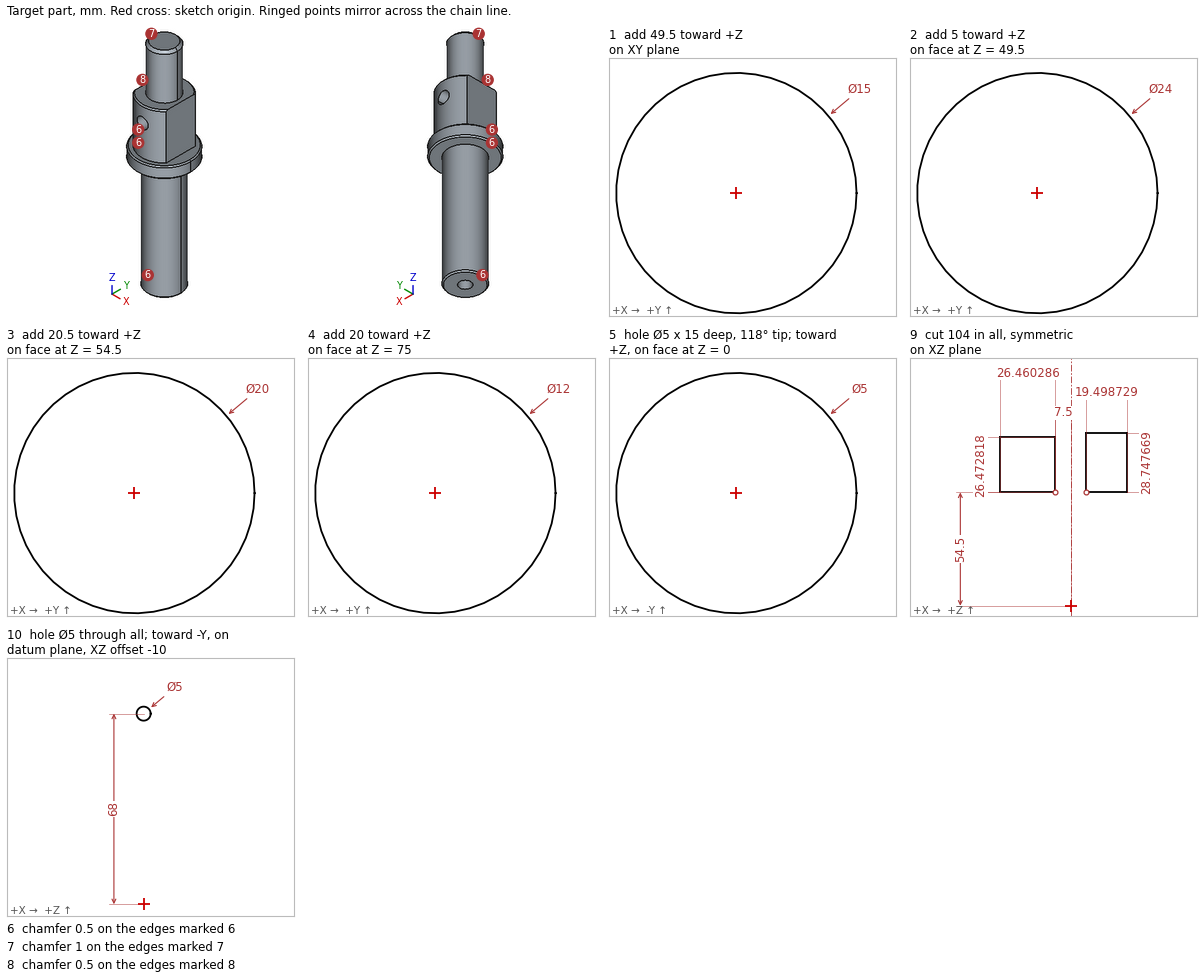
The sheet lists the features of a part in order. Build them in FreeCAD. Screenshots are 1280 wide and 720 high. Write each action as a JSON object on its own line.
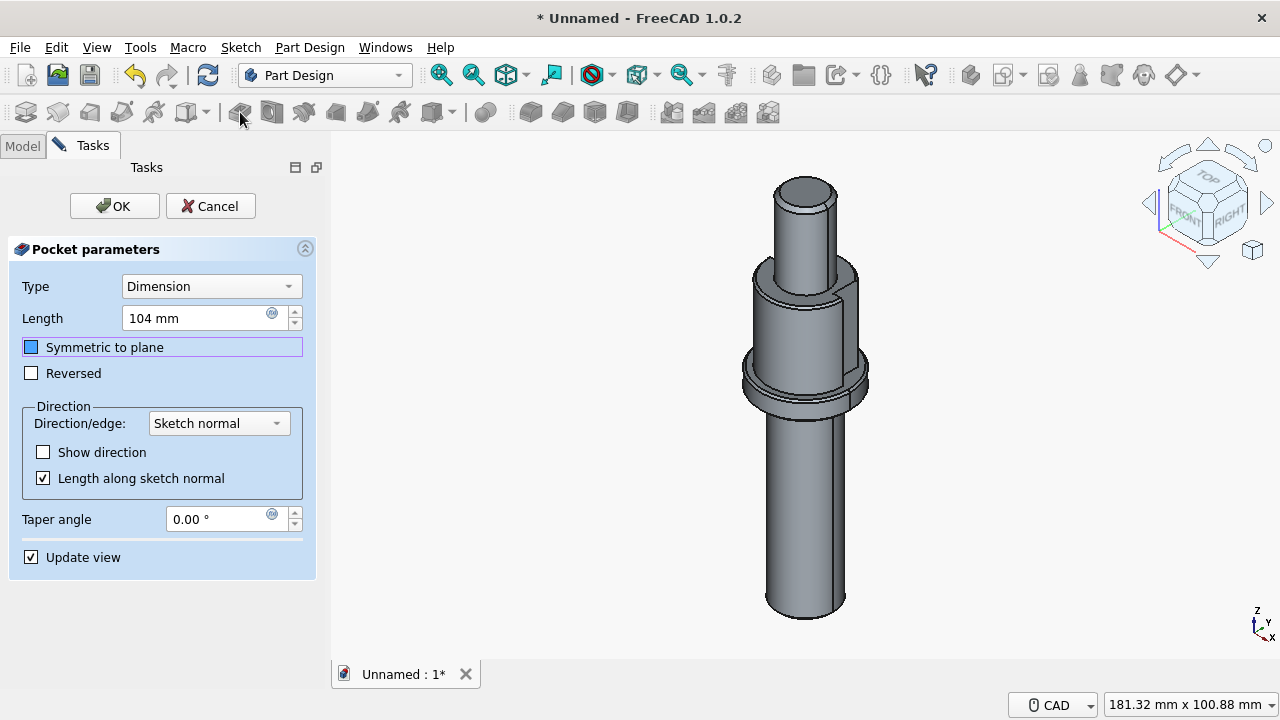
{"action": "left_click", "coordinate": [30, 347]}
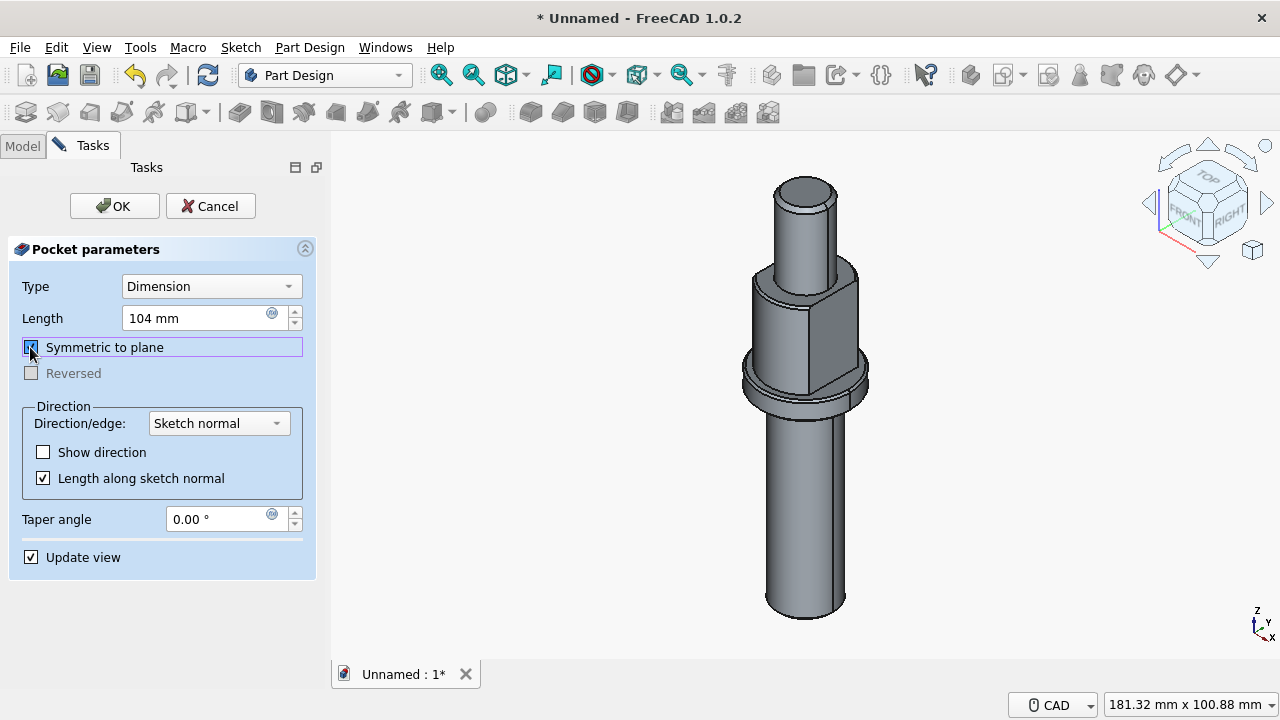
{"action": "left_click", "coordinate": [115, 206]}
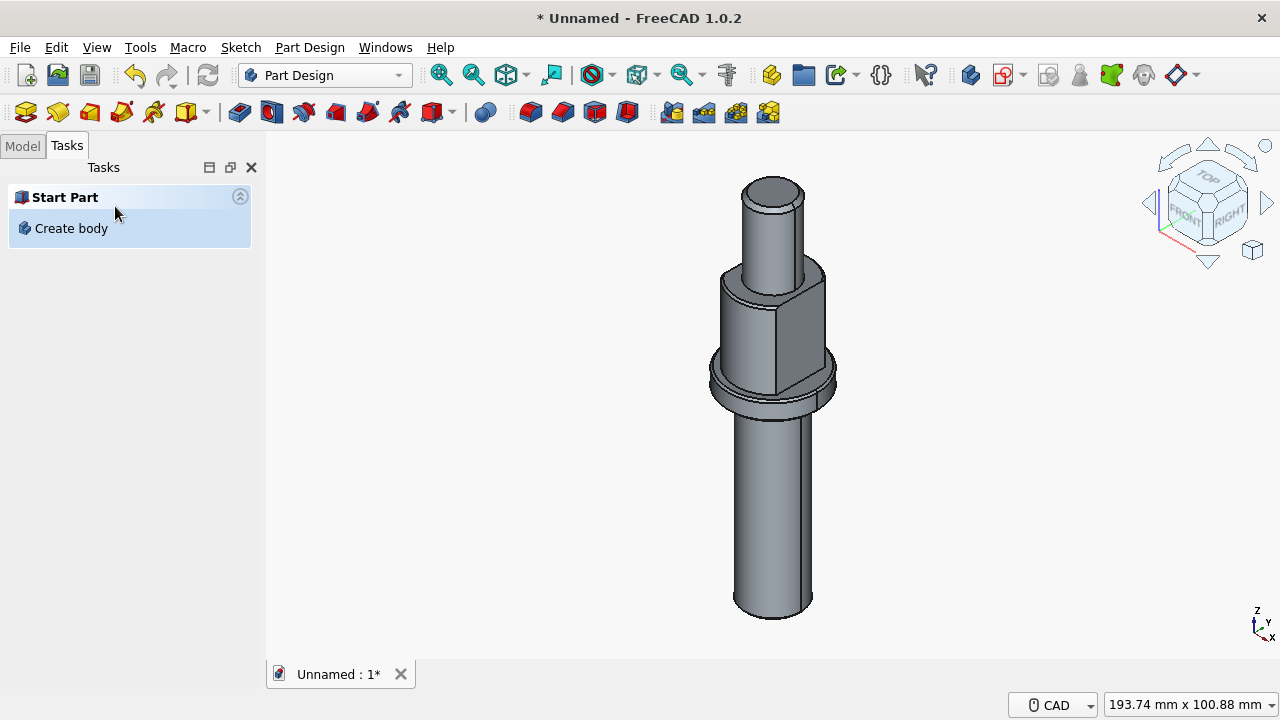
{"action": "left_click", "coordinate": [23, 145]}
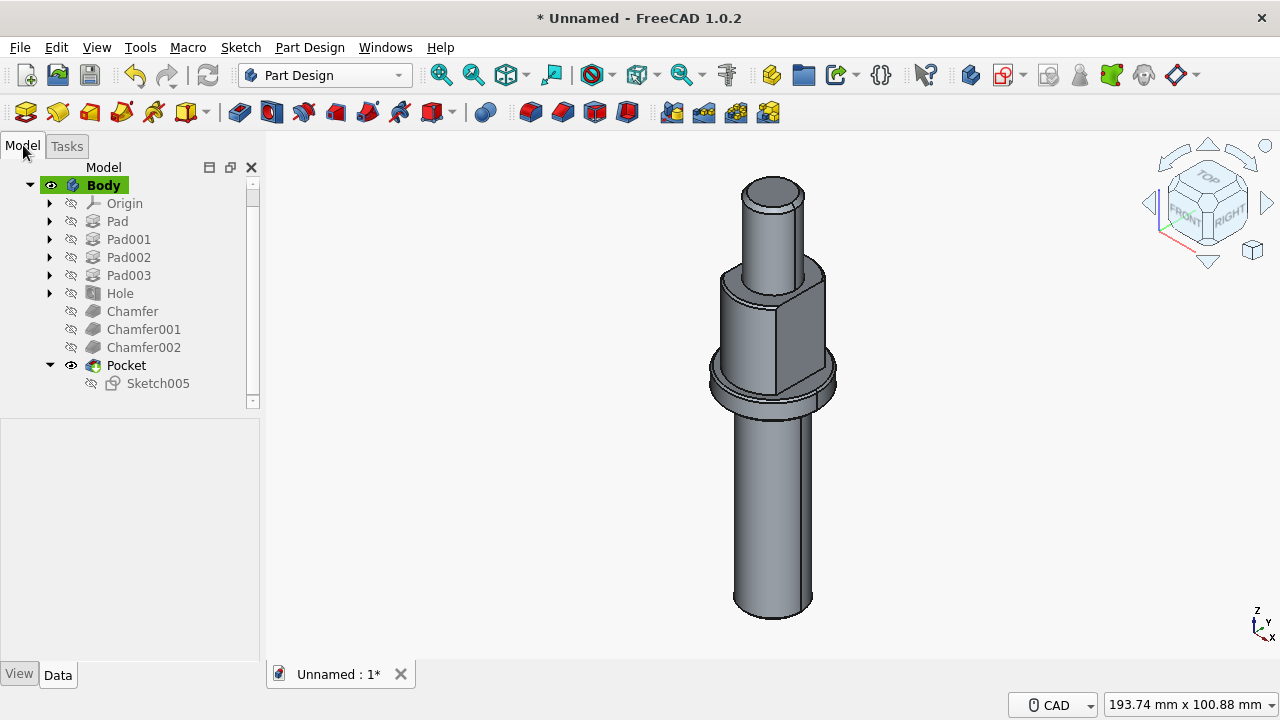
{"action": "left_click", "coordinate": [50, 203]}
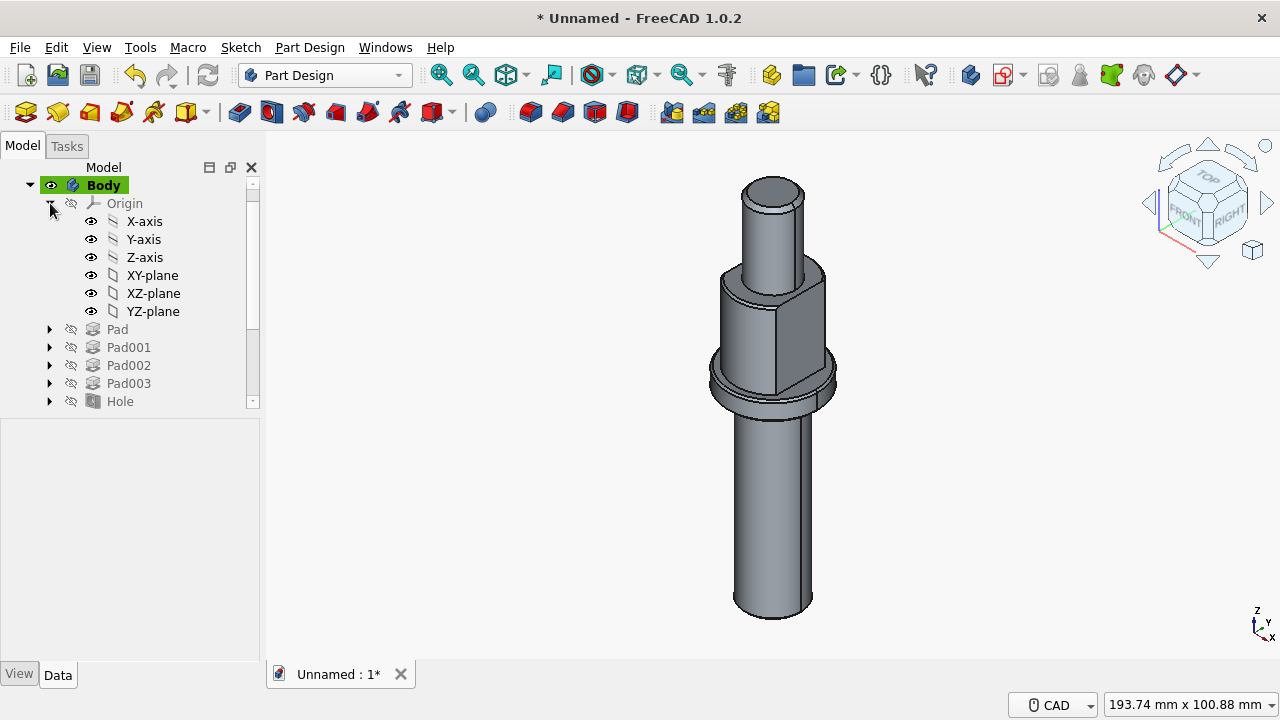
{"action": "left_click", "coordinate": [136, 293]}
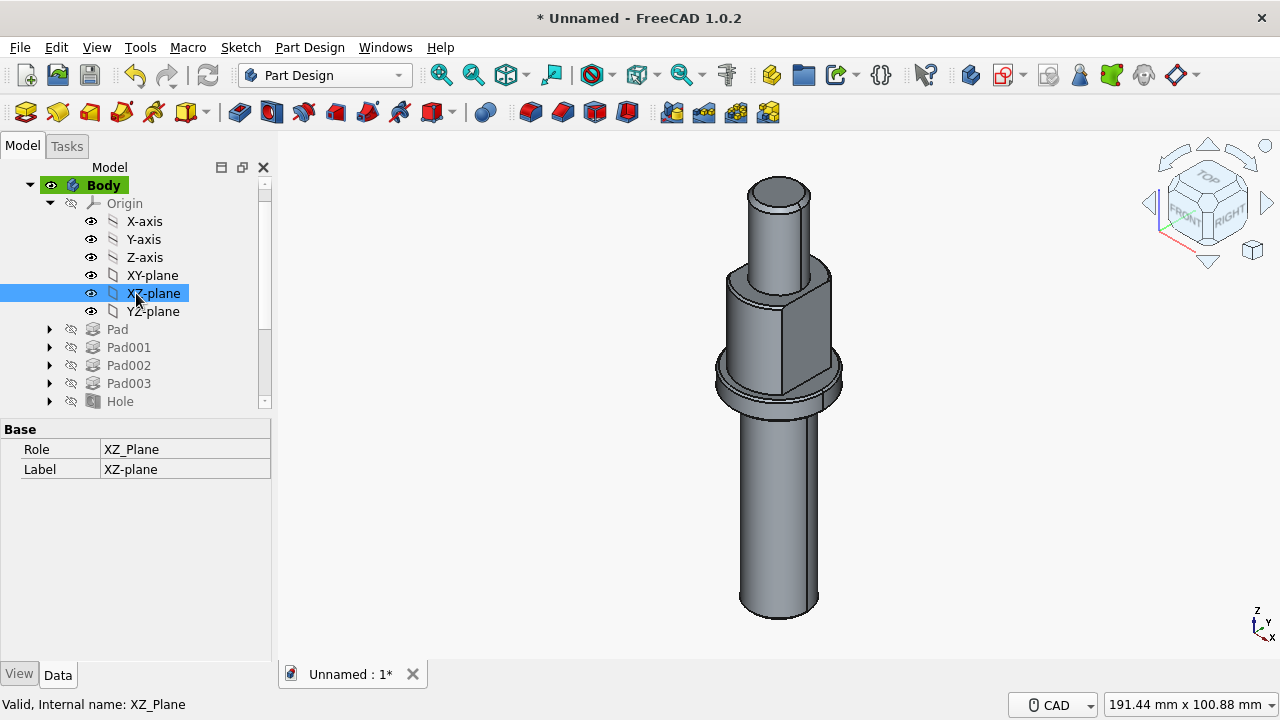
{"action": "left_click", "coordinate": [1176, 76]}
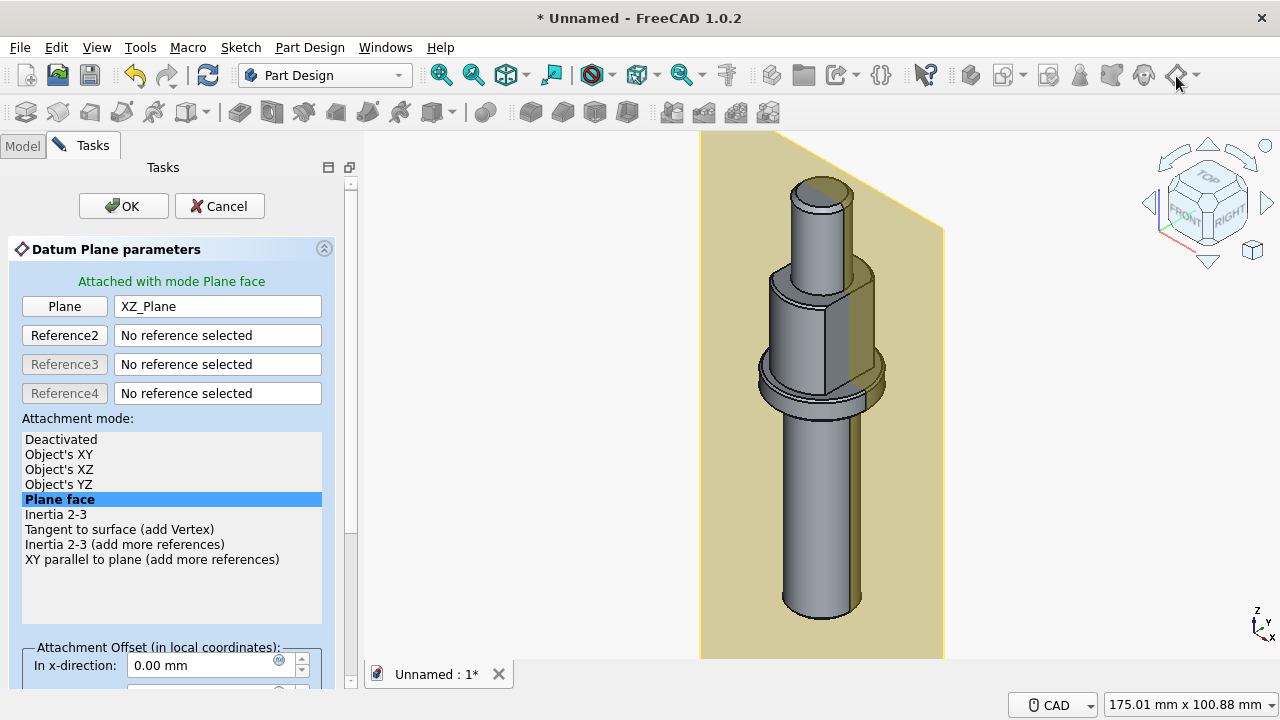
{"action": "scroll", "coordinate": [351, 432], "scroll_direction": "down", "scroll_amount": 2}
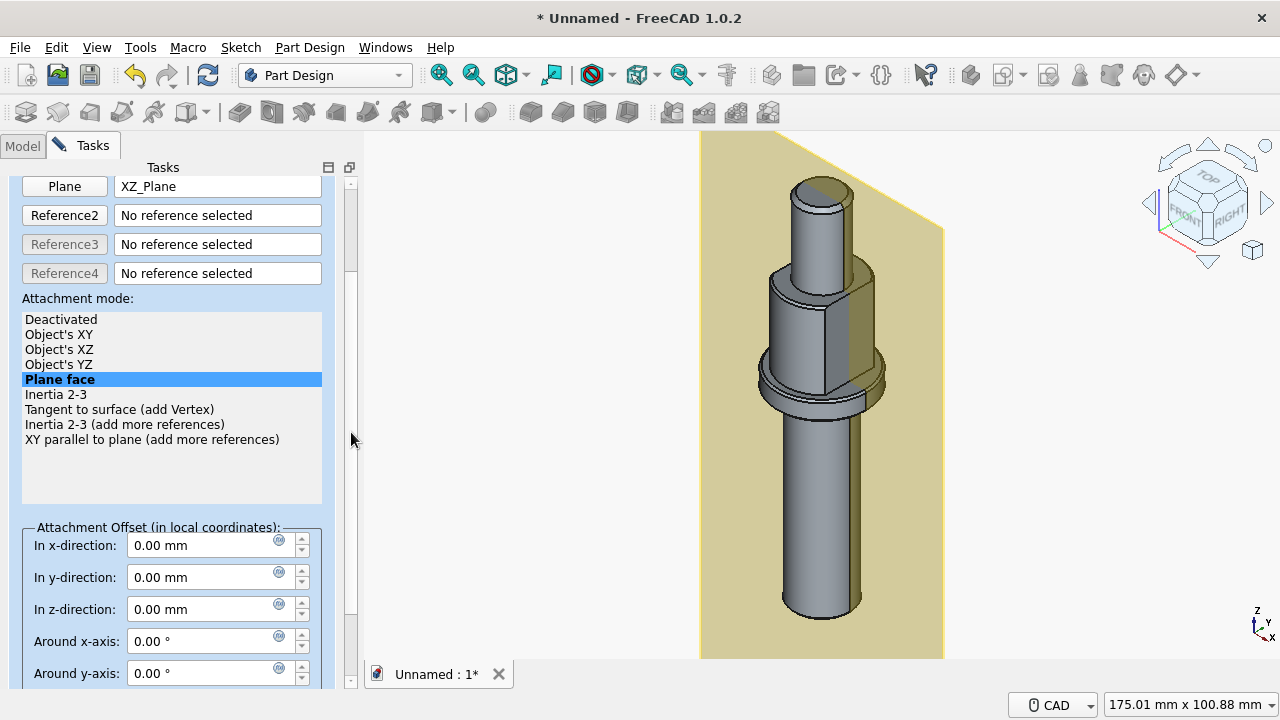
{"action": "triple_click", "coordinate": [210, 609]}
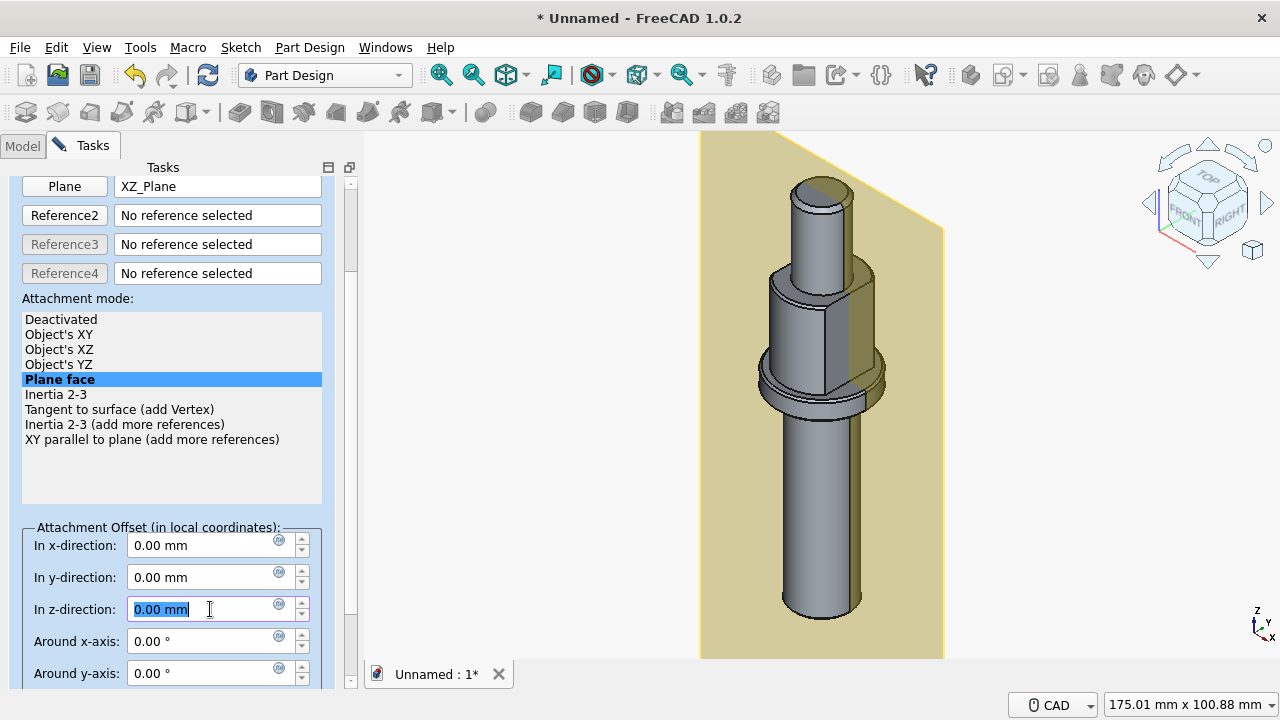
{"action": "type", "text": "-10"}
{"action": "key", "text": "Tab"}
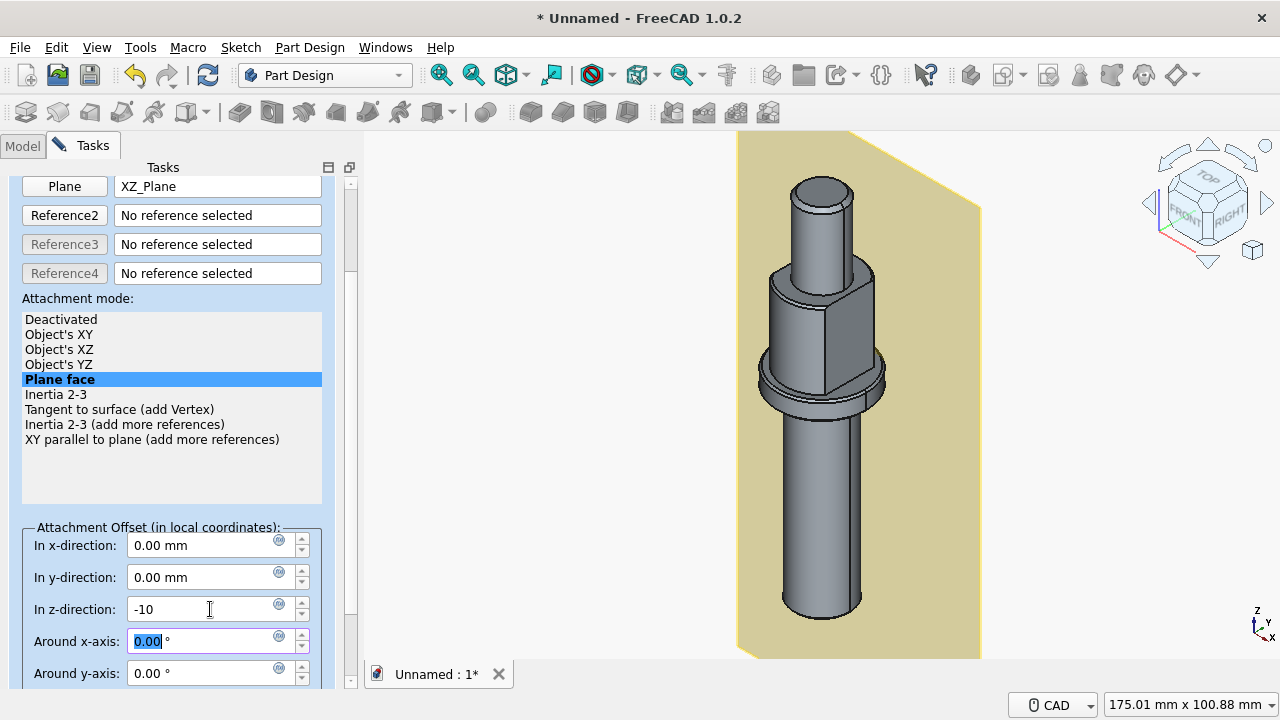
{"action": "scroll", "coordinate": [351, 432], "scroll_direction": "up", "scroll_amount": 3}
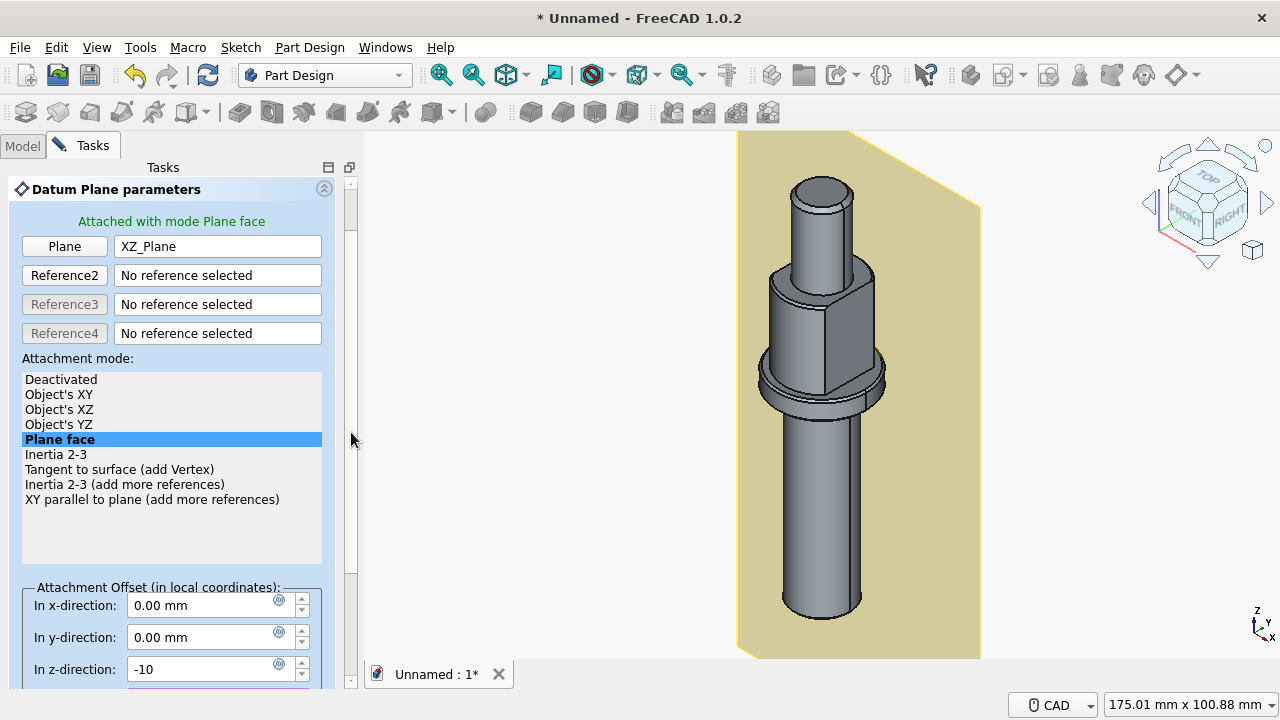
{"action": "left_click", "coordinate": [124, 206]}